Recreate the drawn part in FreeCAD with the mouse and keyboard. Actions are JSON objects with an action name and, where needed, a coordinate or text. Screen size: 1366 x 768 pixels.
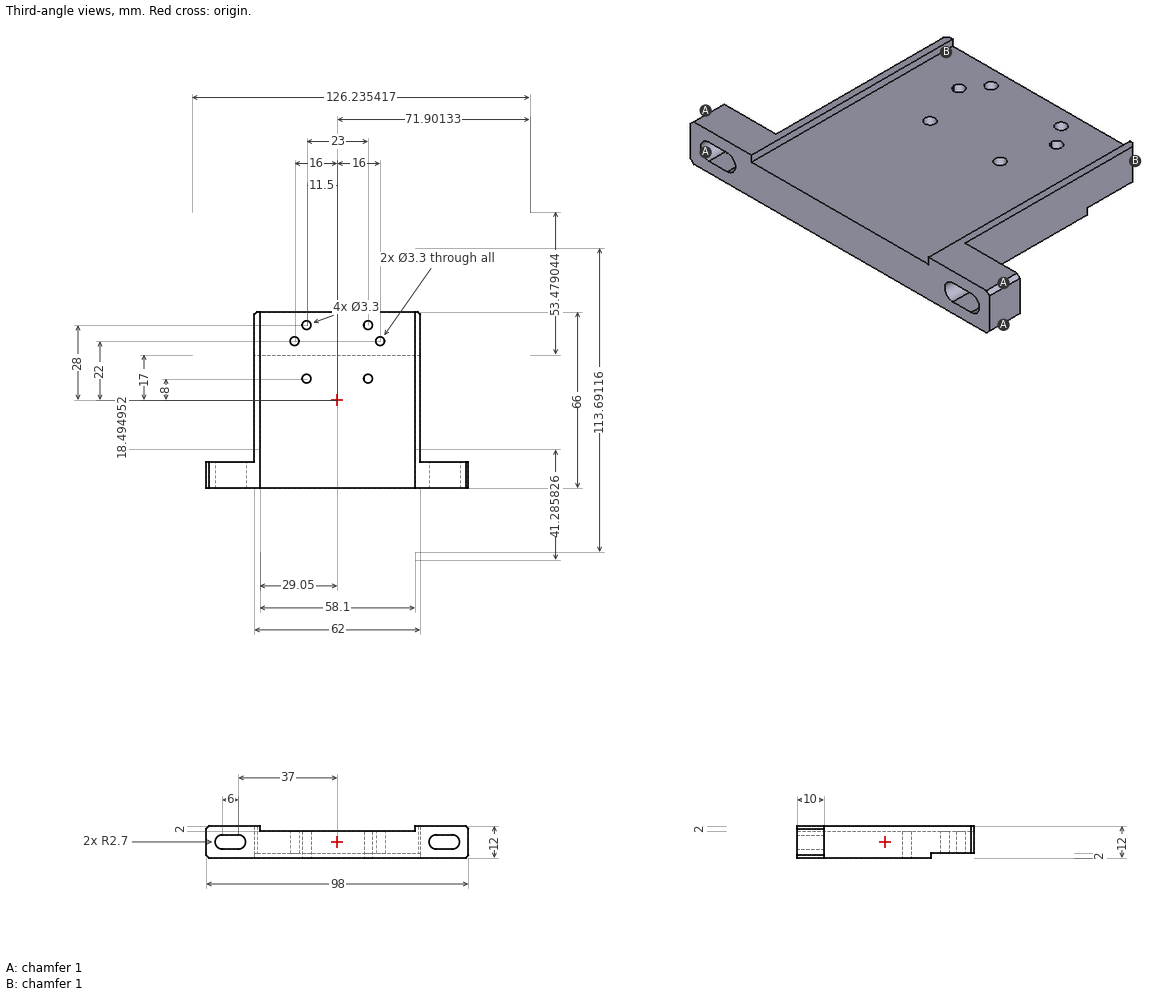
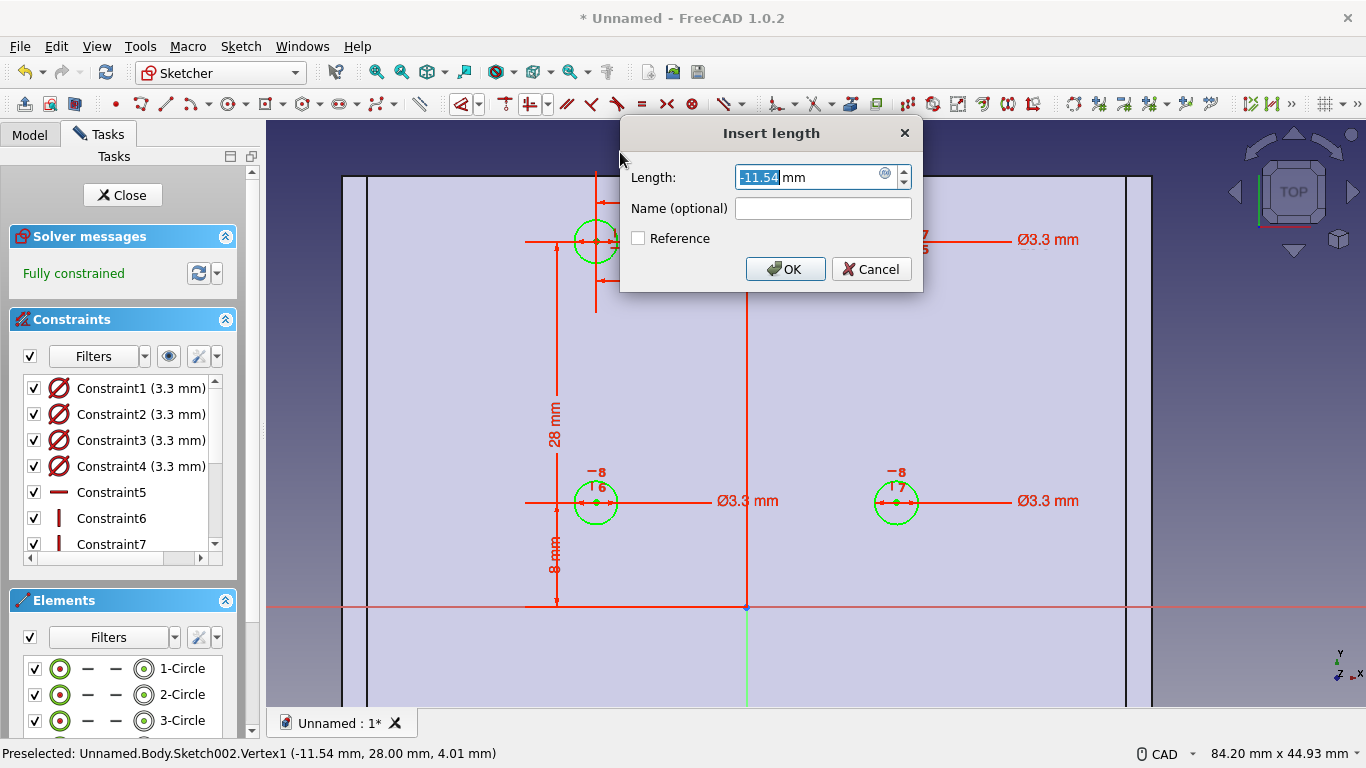
{"action": "type", "text": "-11.5"}
{"action": "key", "text": "Return"}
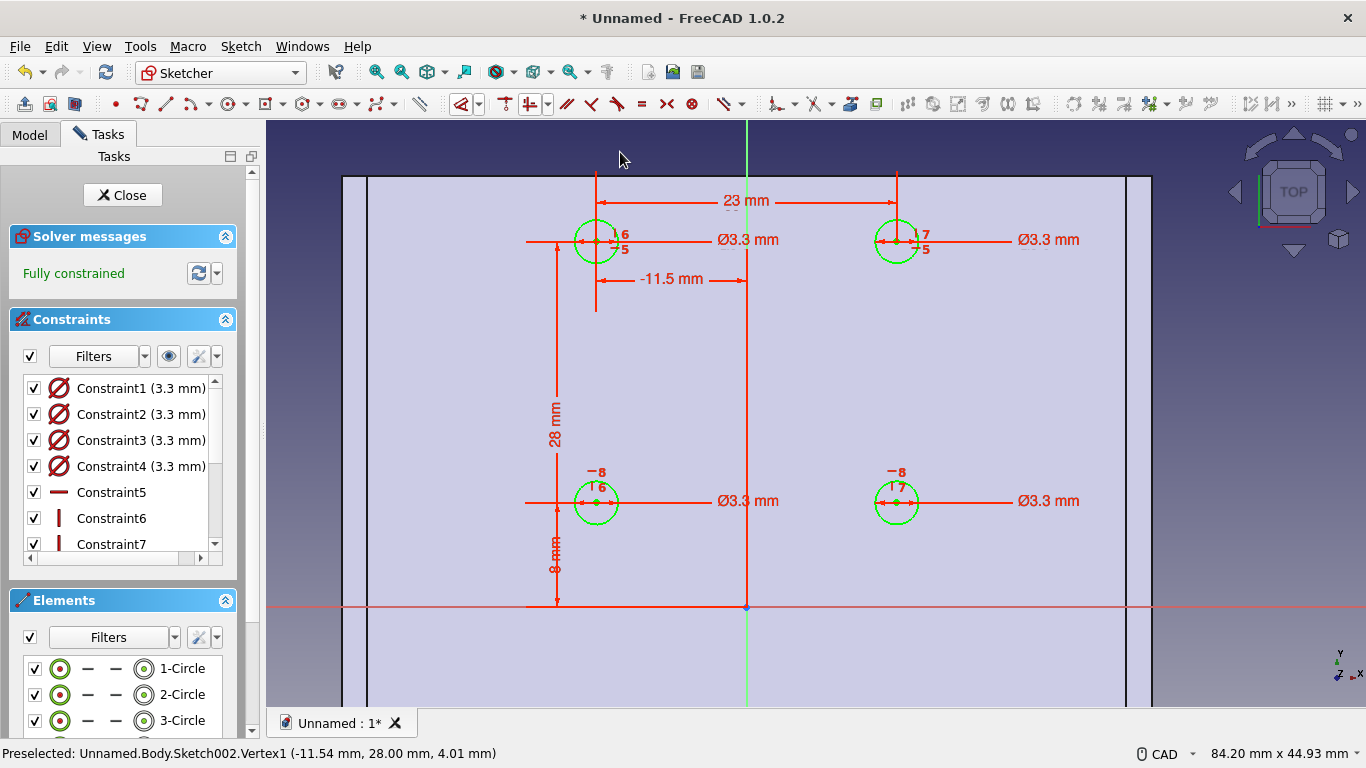
{"action": "left_click", "coordinate": [123, 195]}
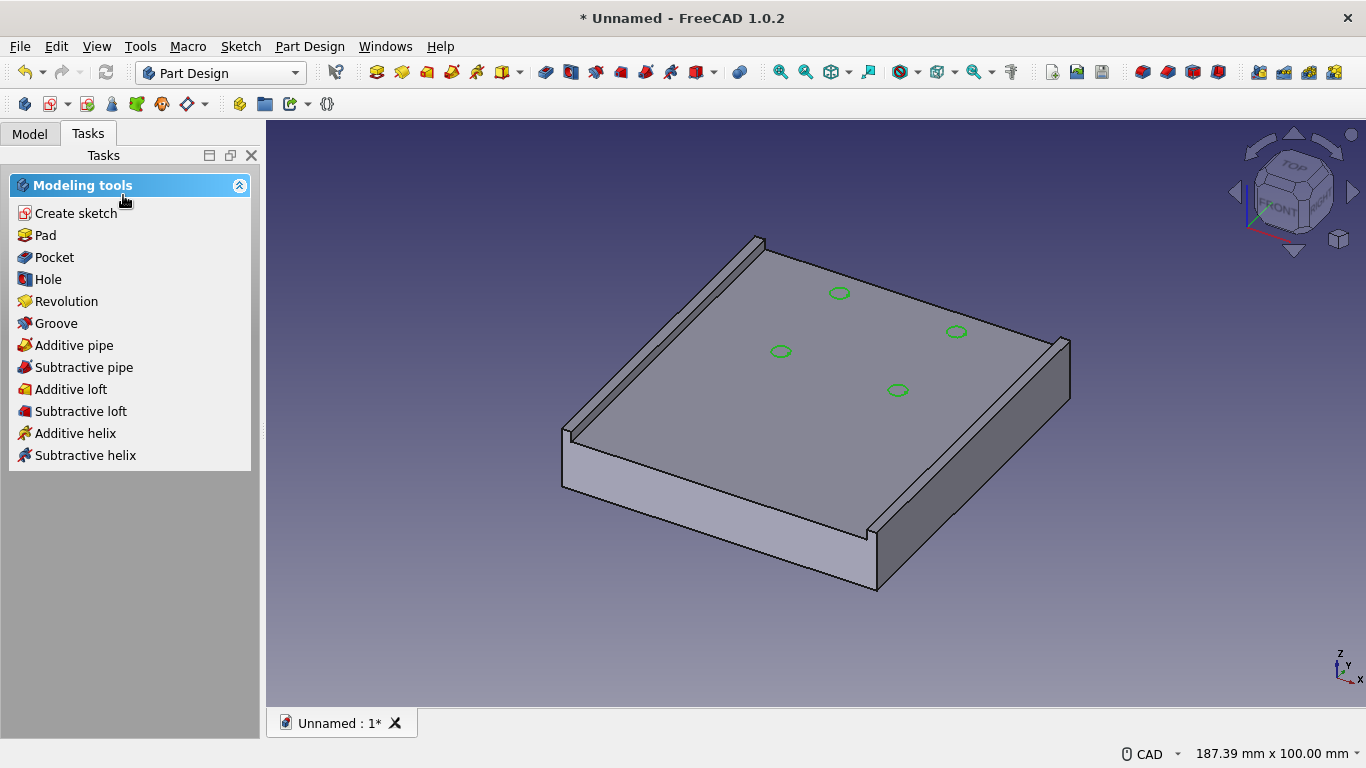
{"action": "left_click", "coordinate": [546, 72]}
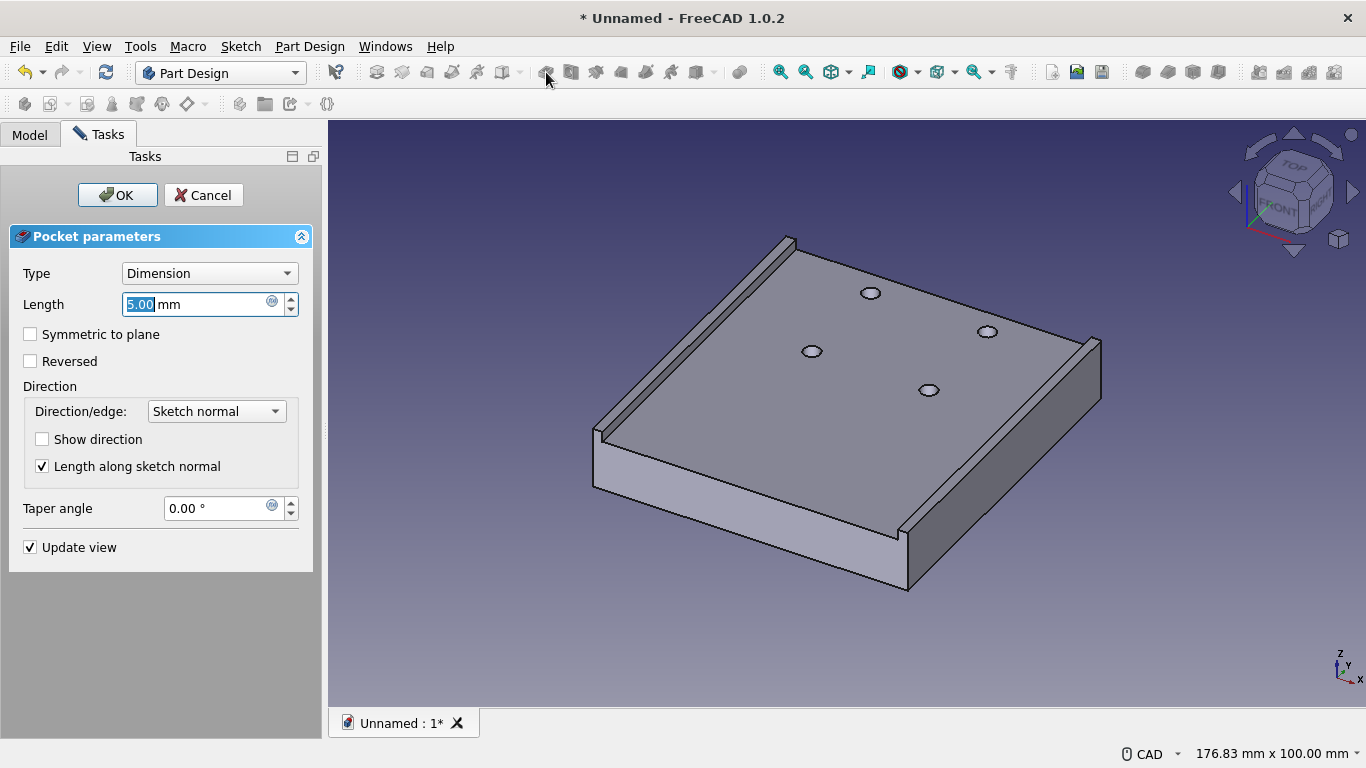
{"action": "left_click", "coordinate": [210, 274]}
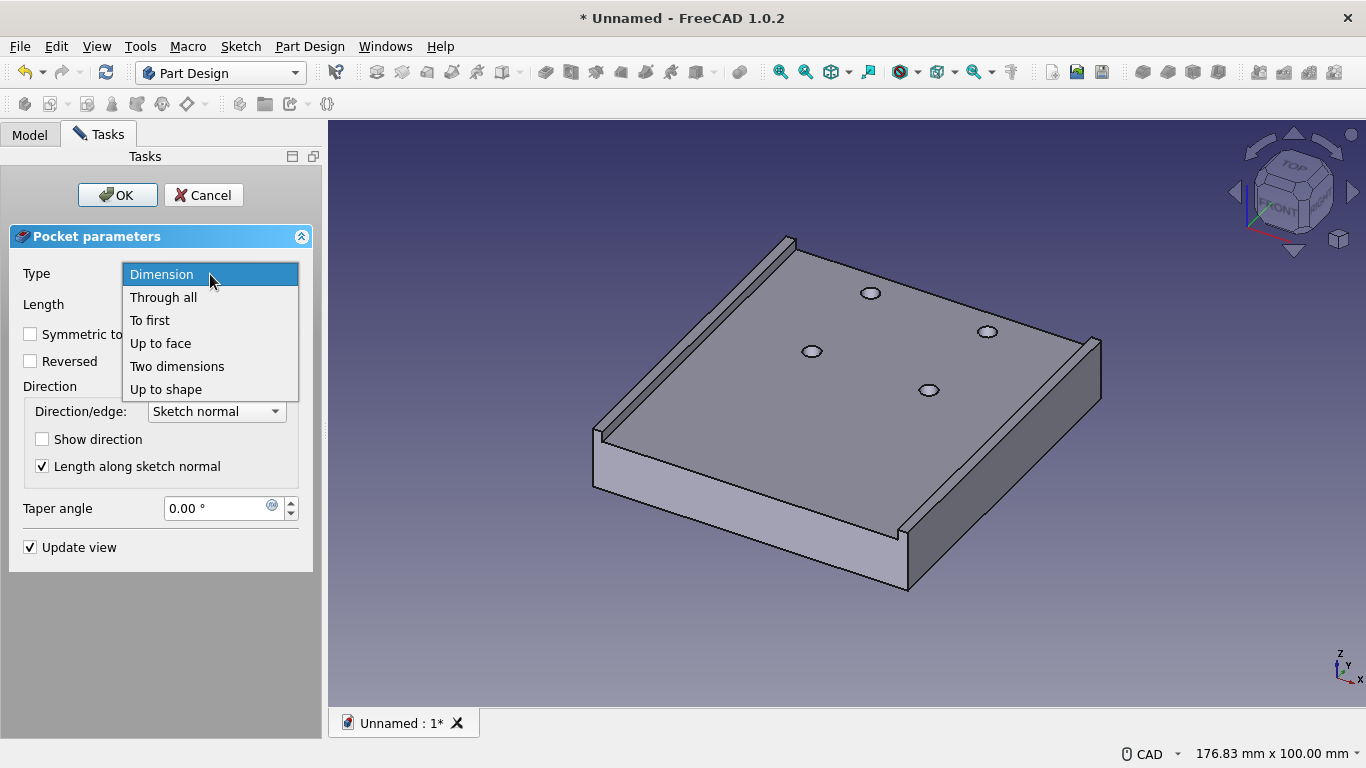
{"action": "left_click", "coordinate": [208, 298]}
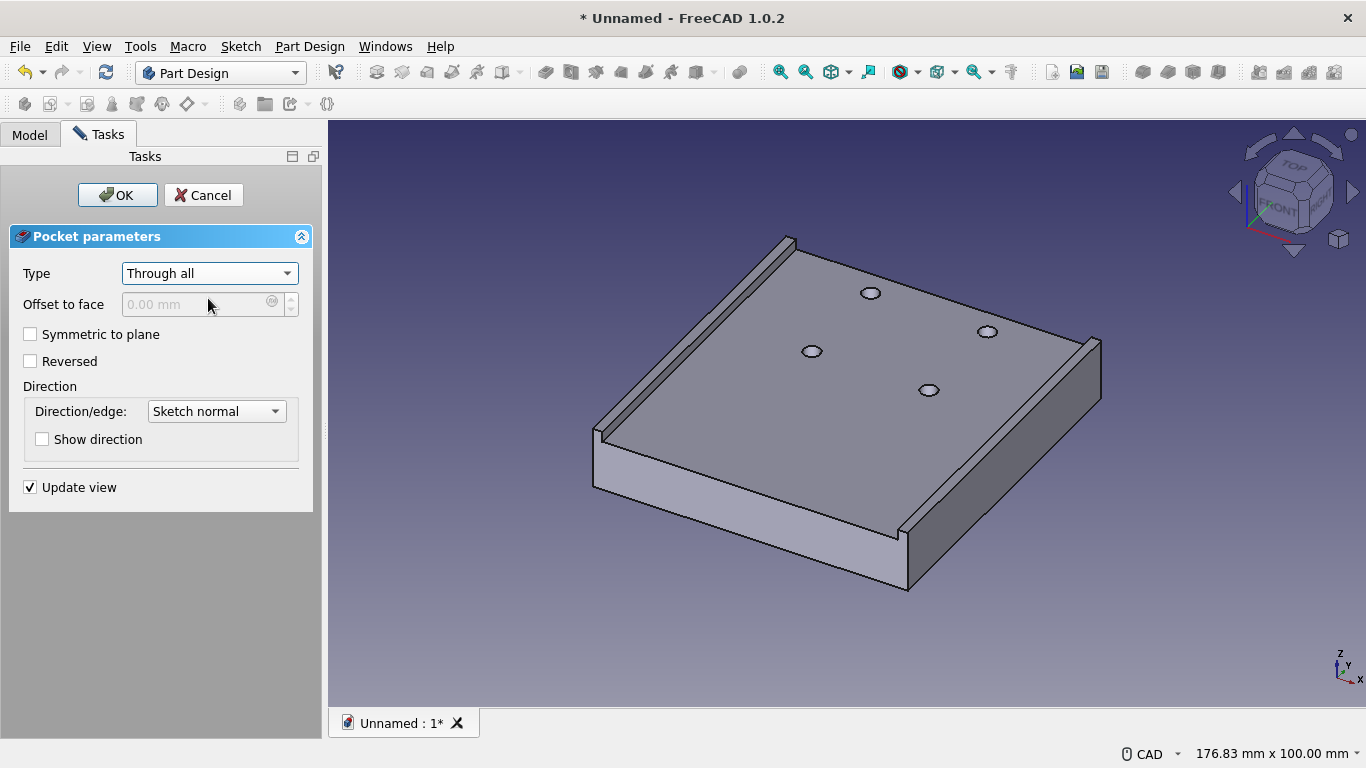
{"action": "left_click", "coordinate": [118, 195]}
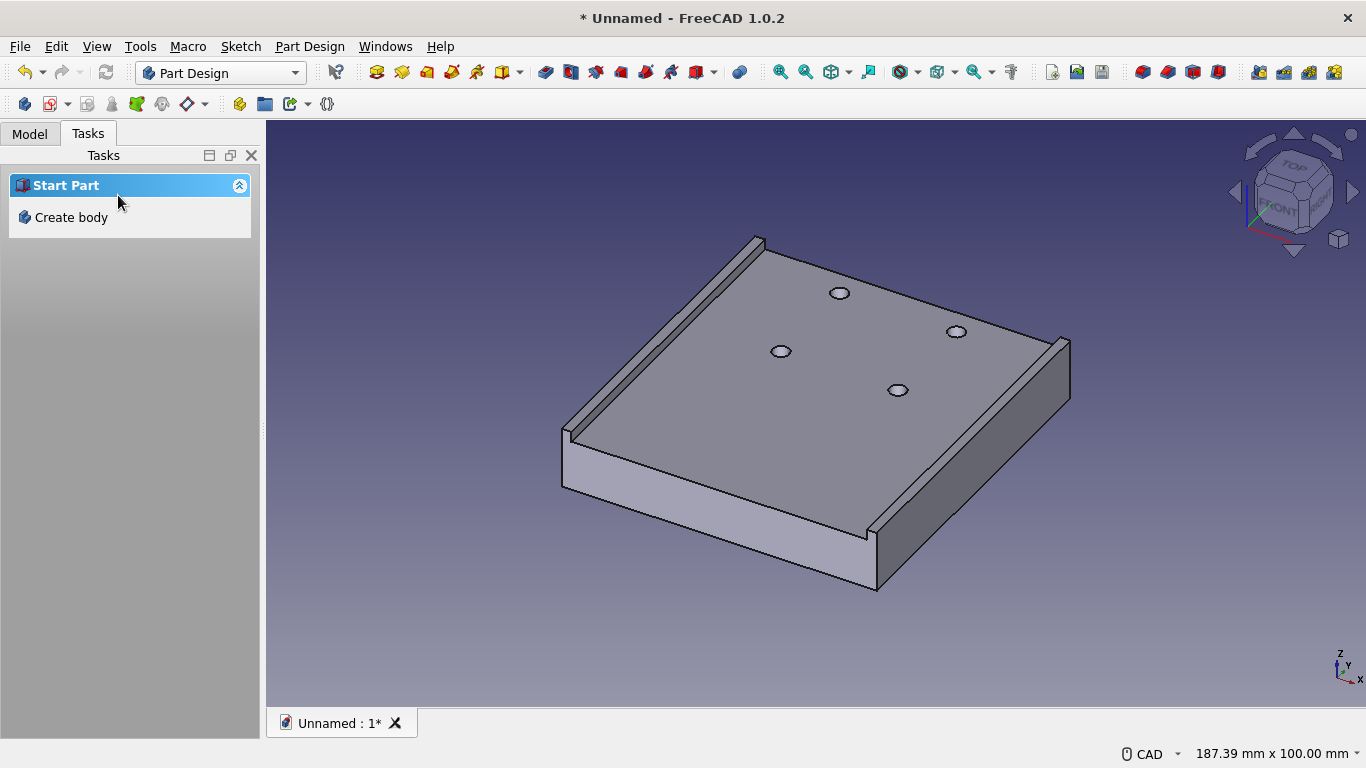
{"action": "key", "text": "5"}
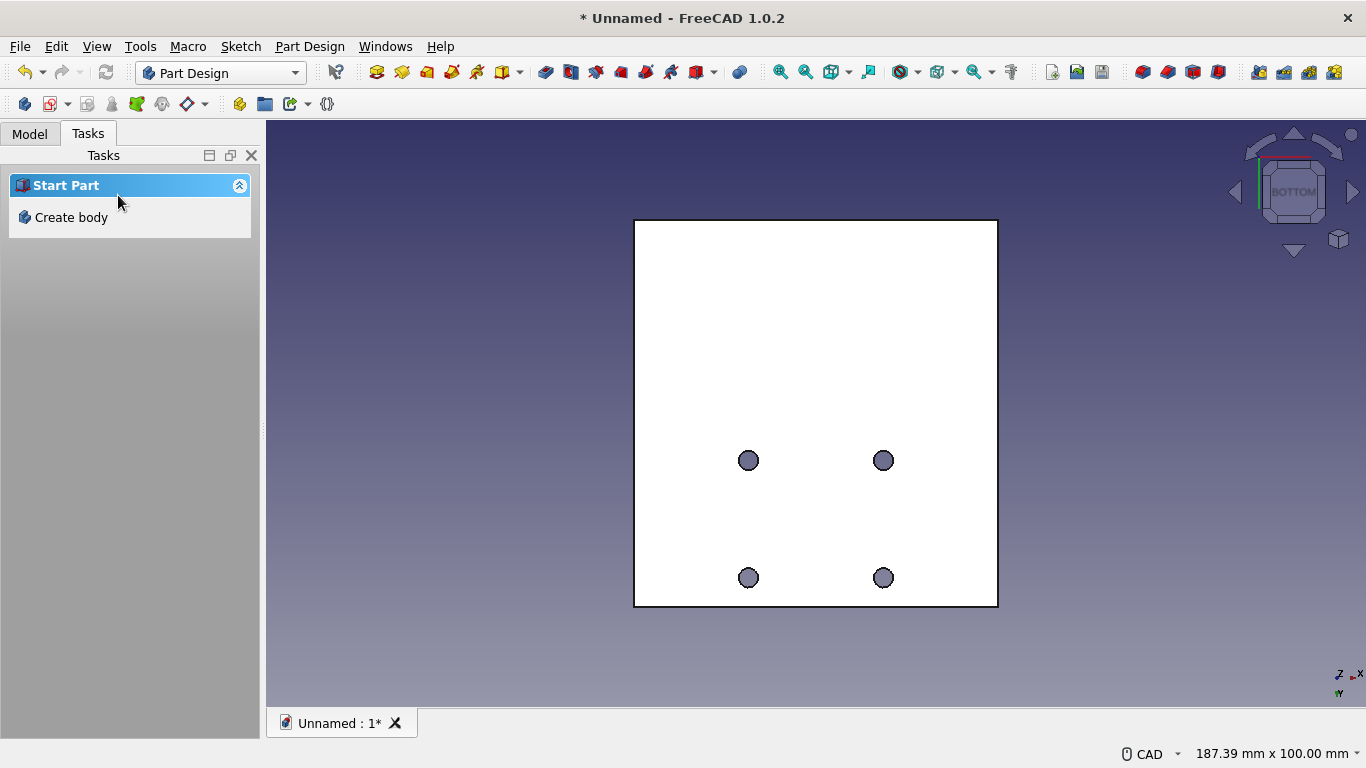
{"action": "left_click", "coordinate": [816, 357]}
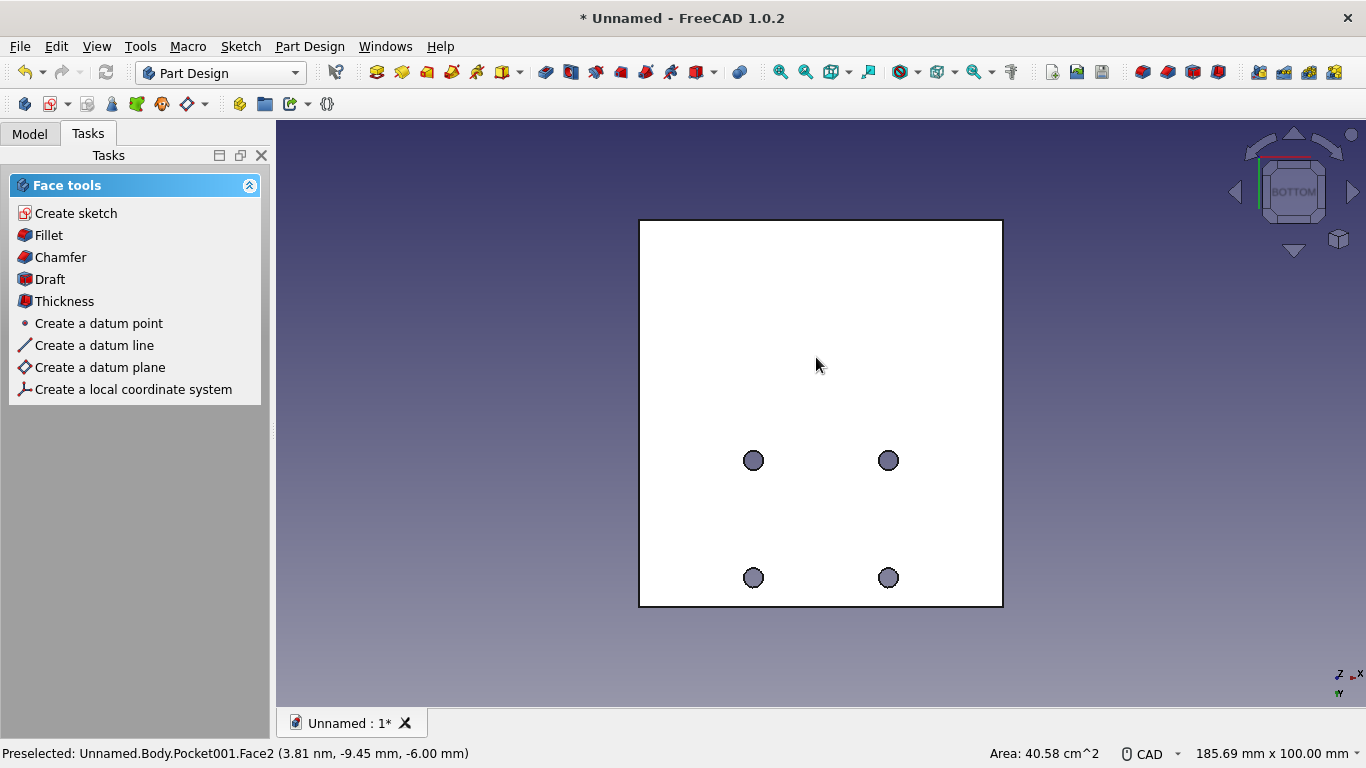
{"action": "left_click", "coordinate": [50, 104]}